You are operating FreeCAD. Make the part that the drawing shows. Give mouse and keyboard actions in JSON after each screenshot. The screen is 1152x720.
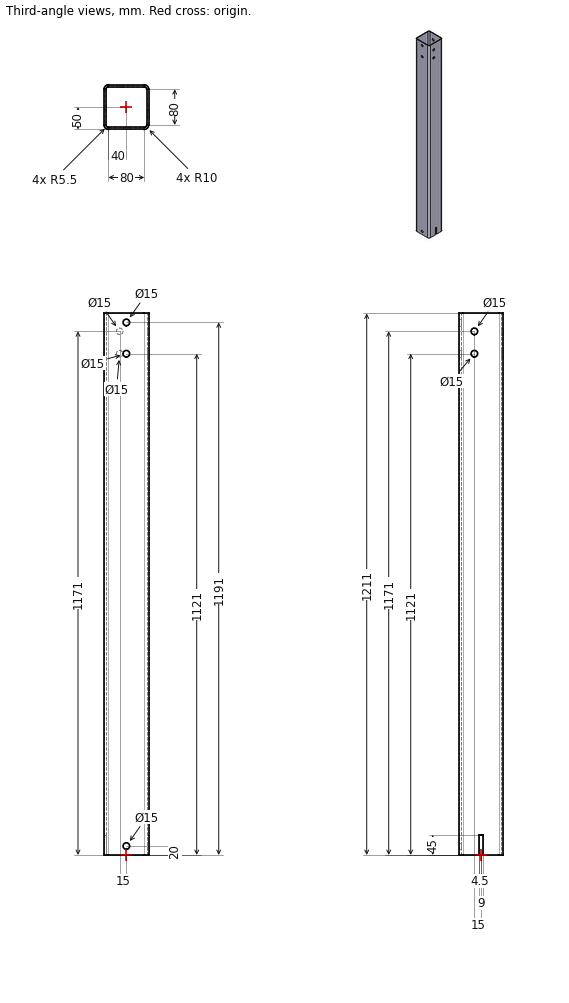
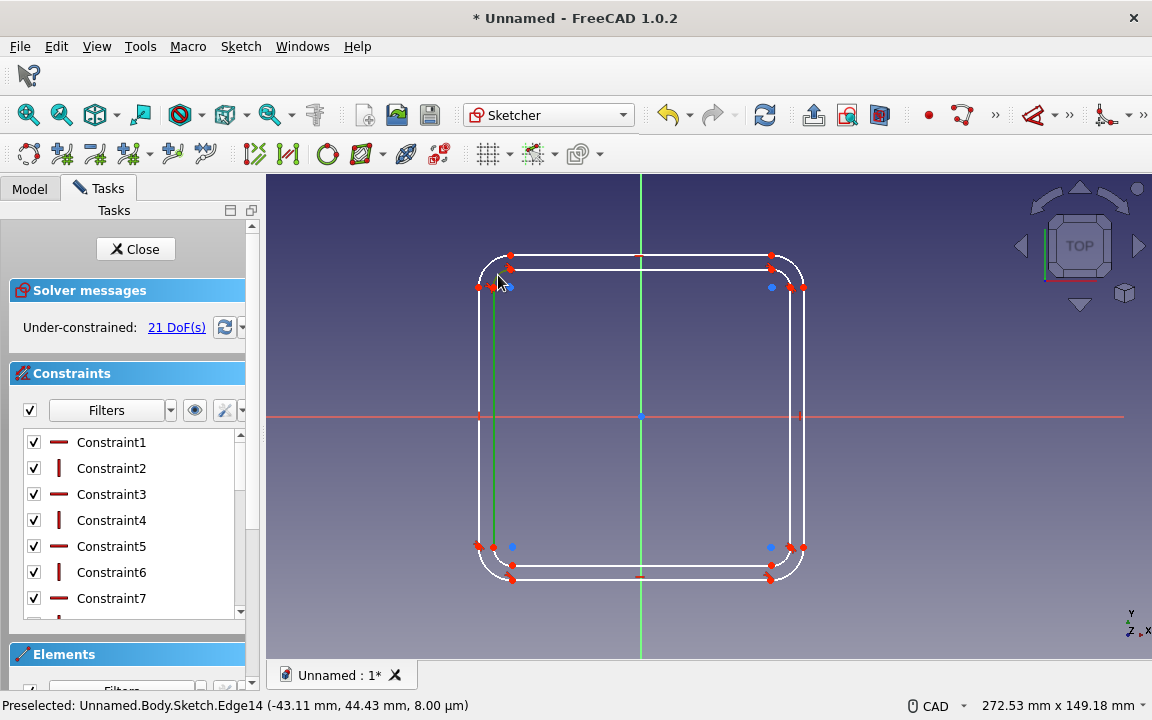
{"action": "key", "text": "t"}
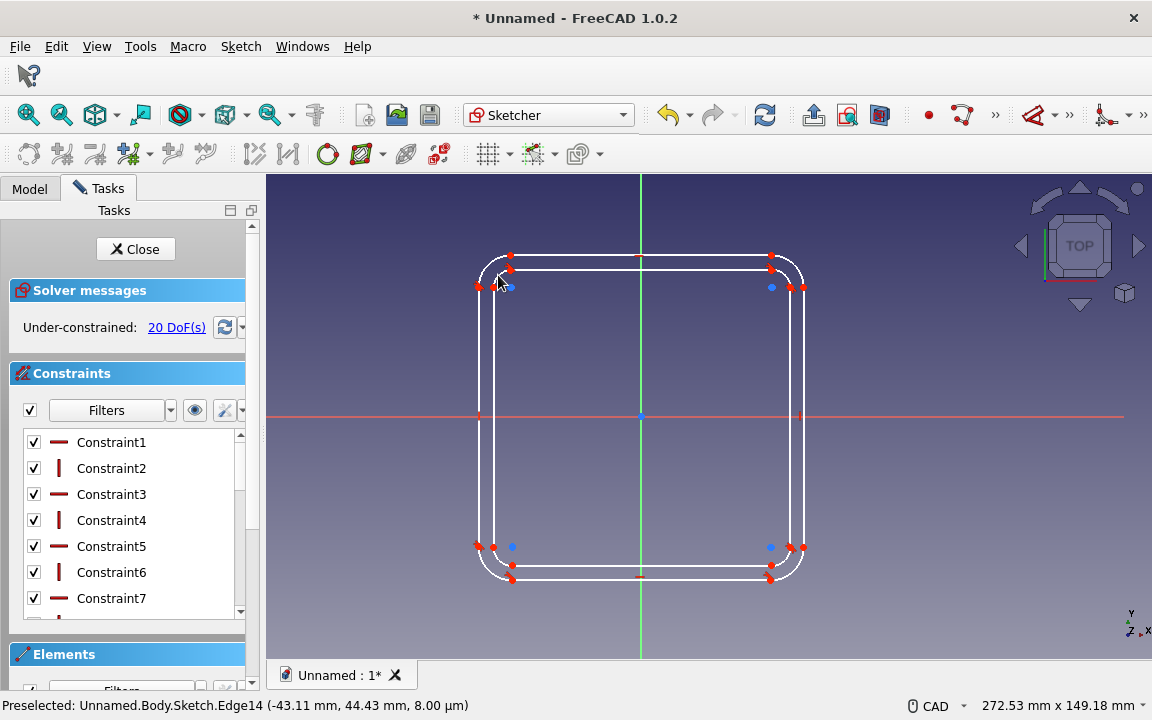
{"action": "left_click", "coordinate": [589, 270]}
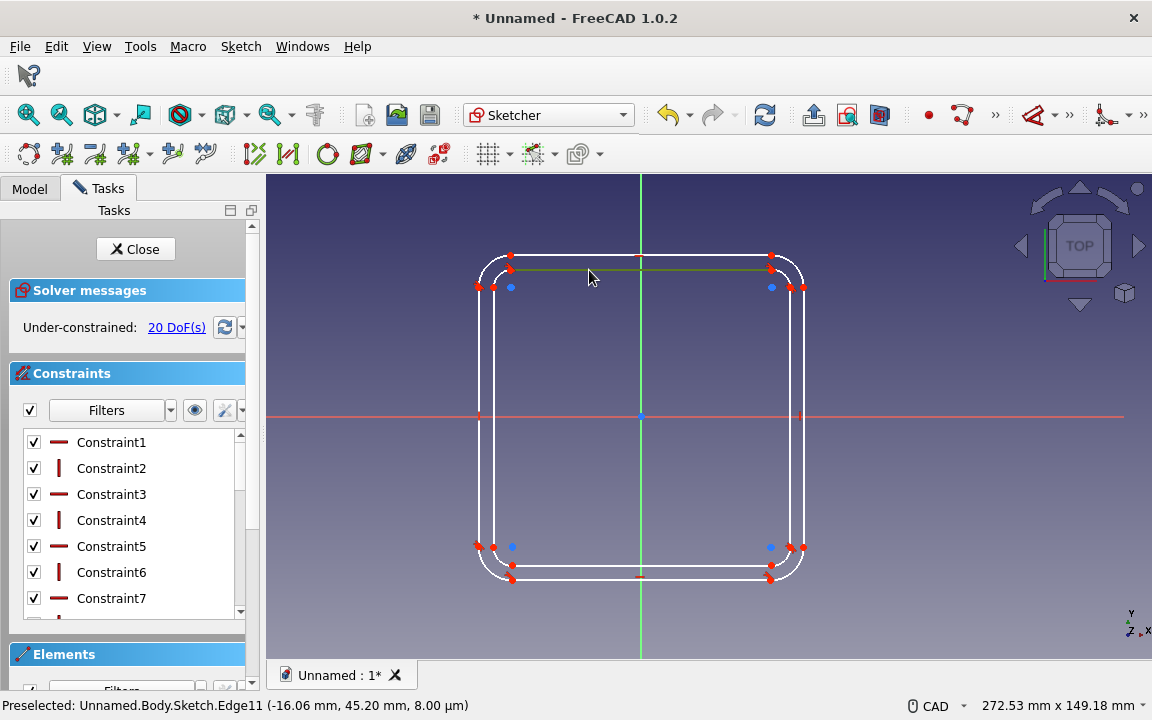
{"action": "left_click", "coordinate": [499, 276]}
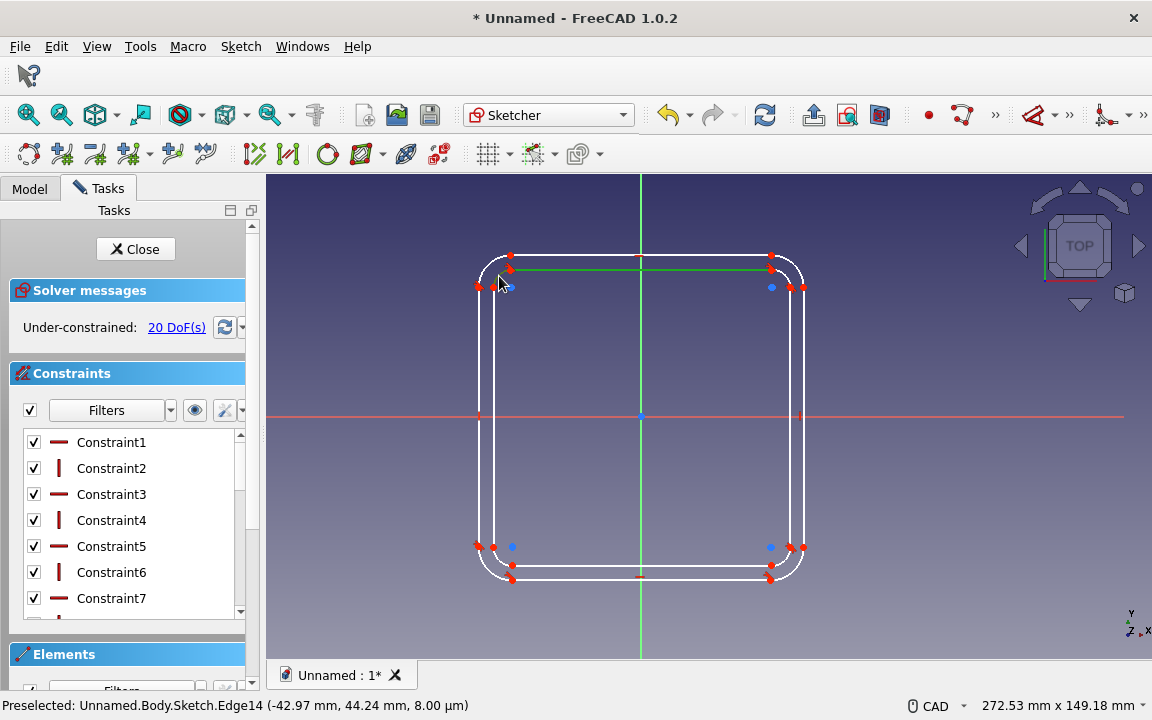
{"action": "key", "text": "t"}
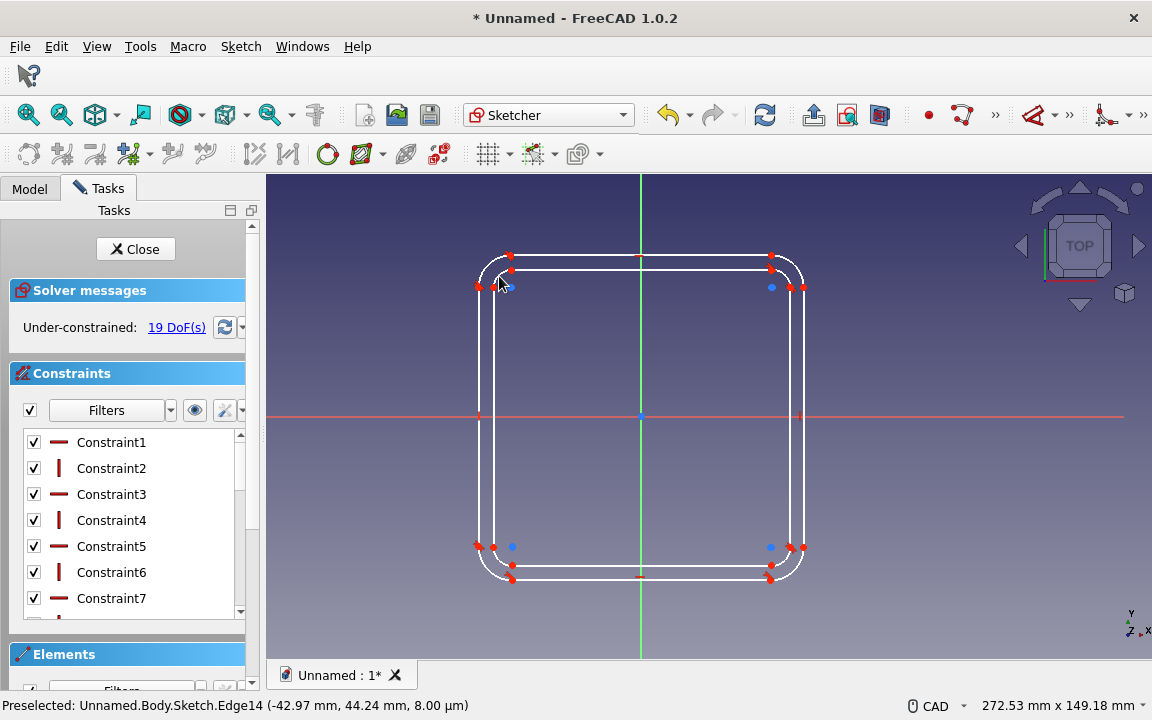
{"action": "left_click", "coordinate": [590, 270]}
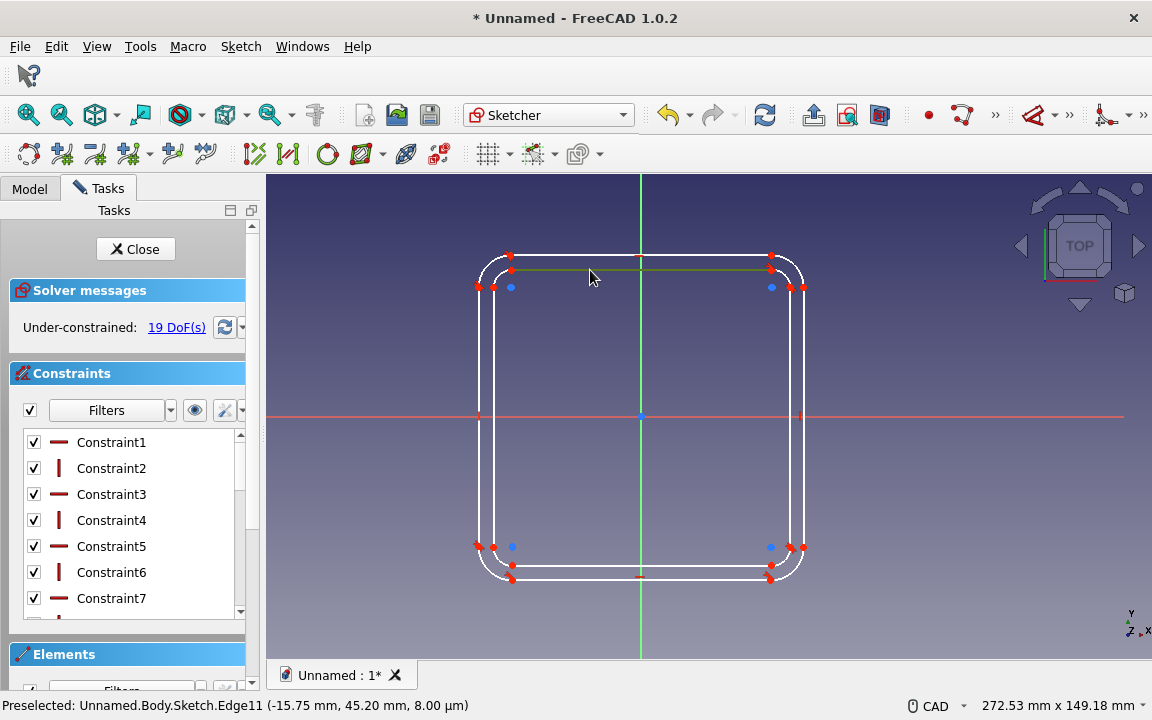
{"action": "left_click", "coordinate": [785, 275]}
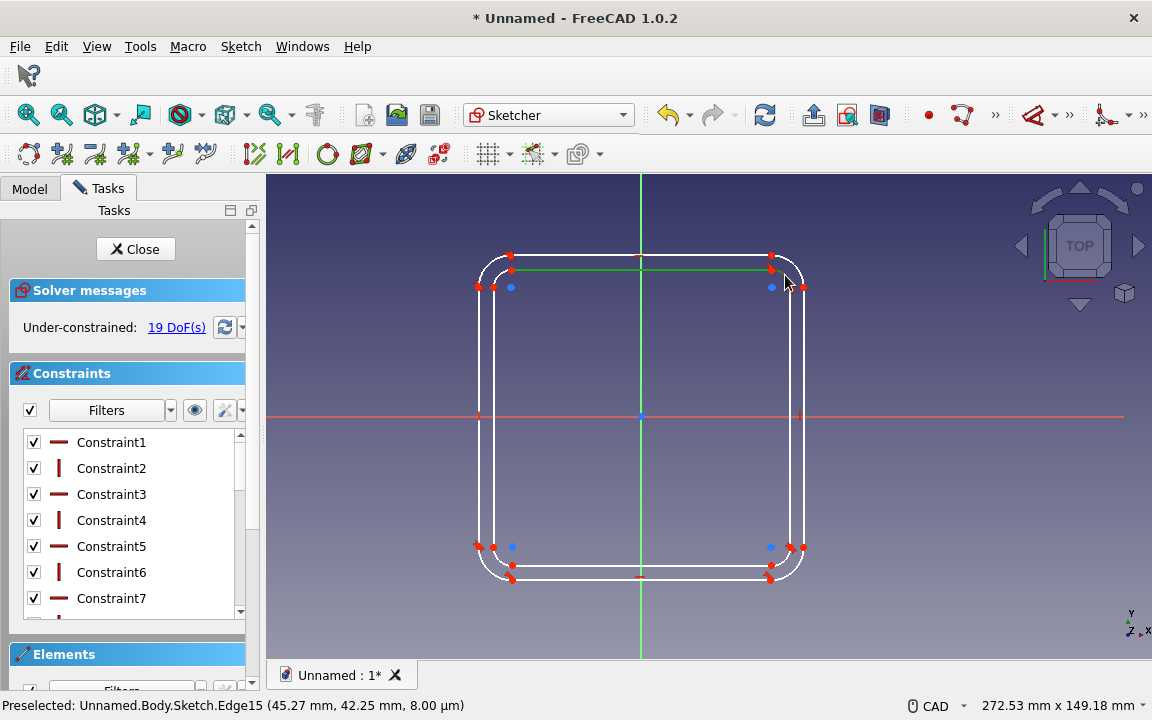
{"action": "key", "text": "t"}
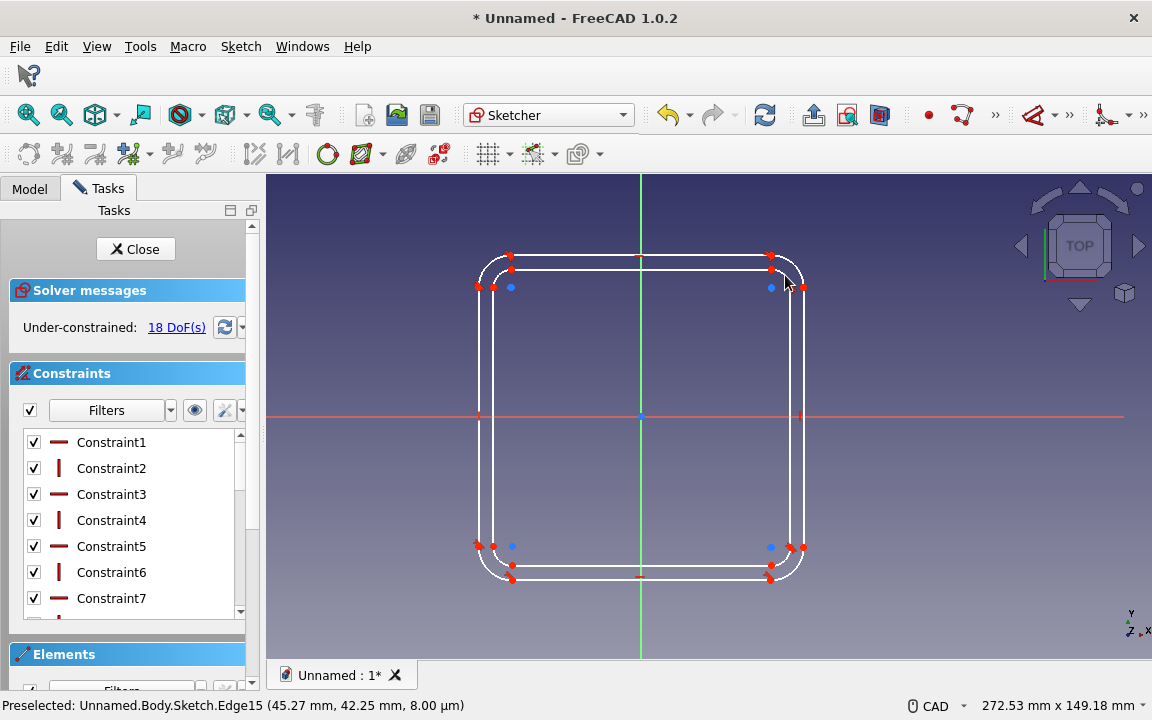
{"action": "left_click", "coordinate": [790, 366]}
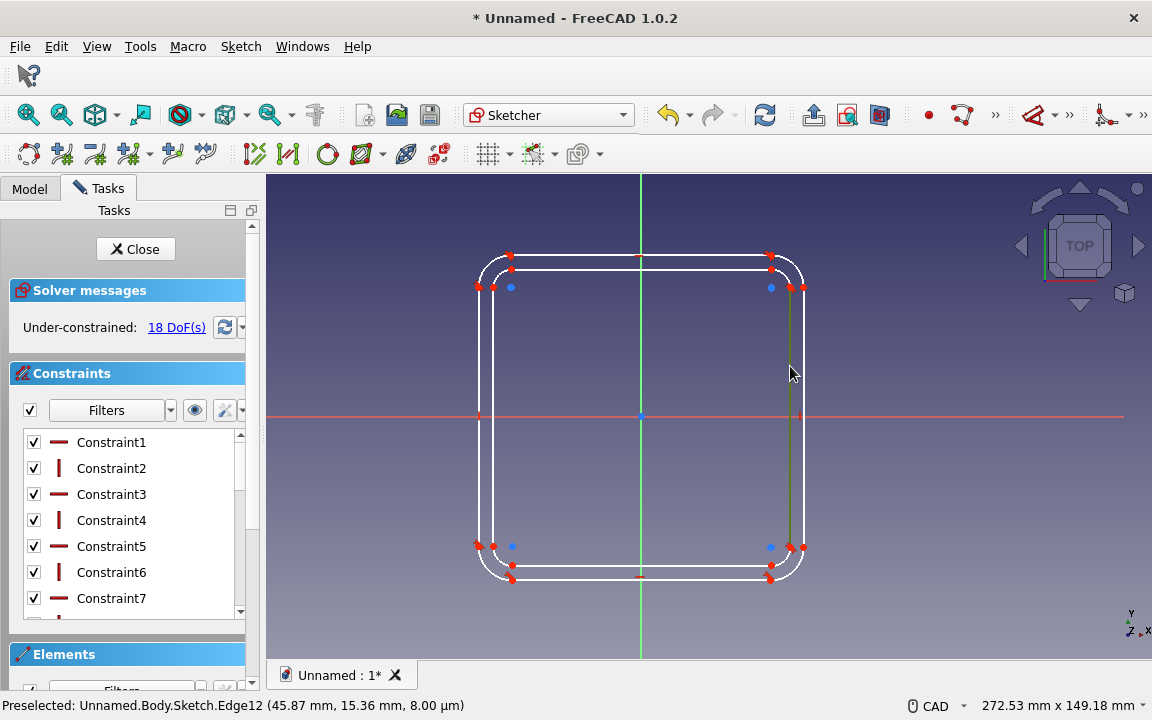
{"action": "left_click", "coordinate": [785, 275]}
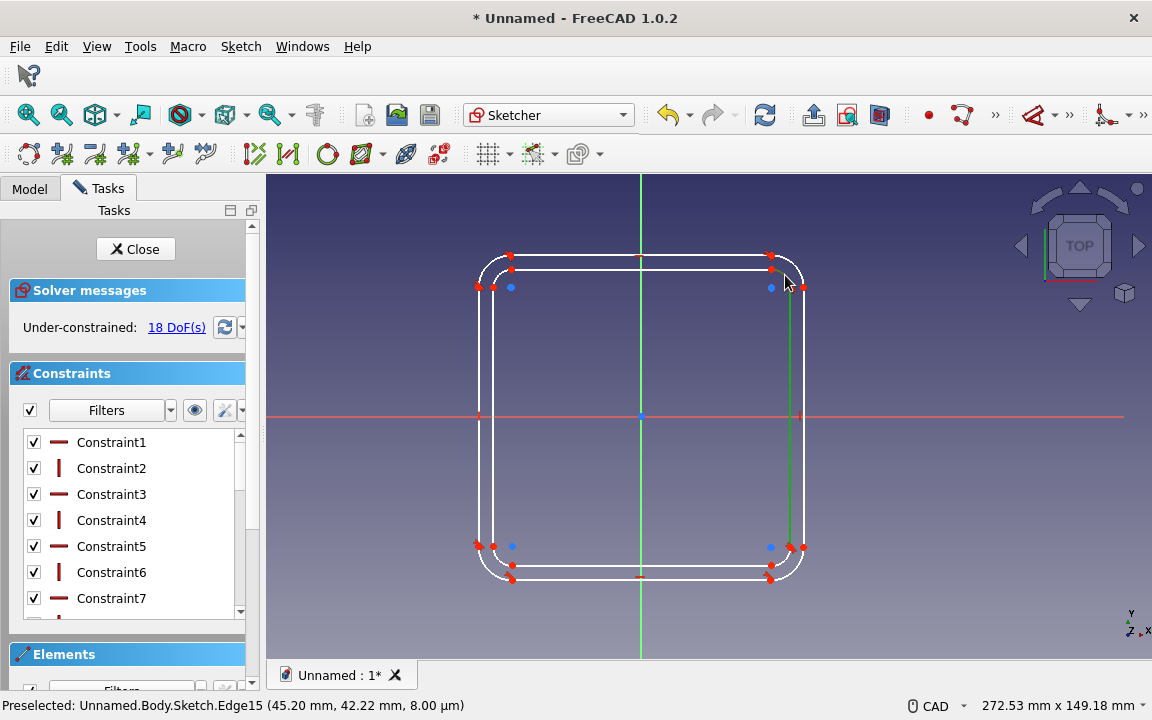
{"action": "key", "text": "t"}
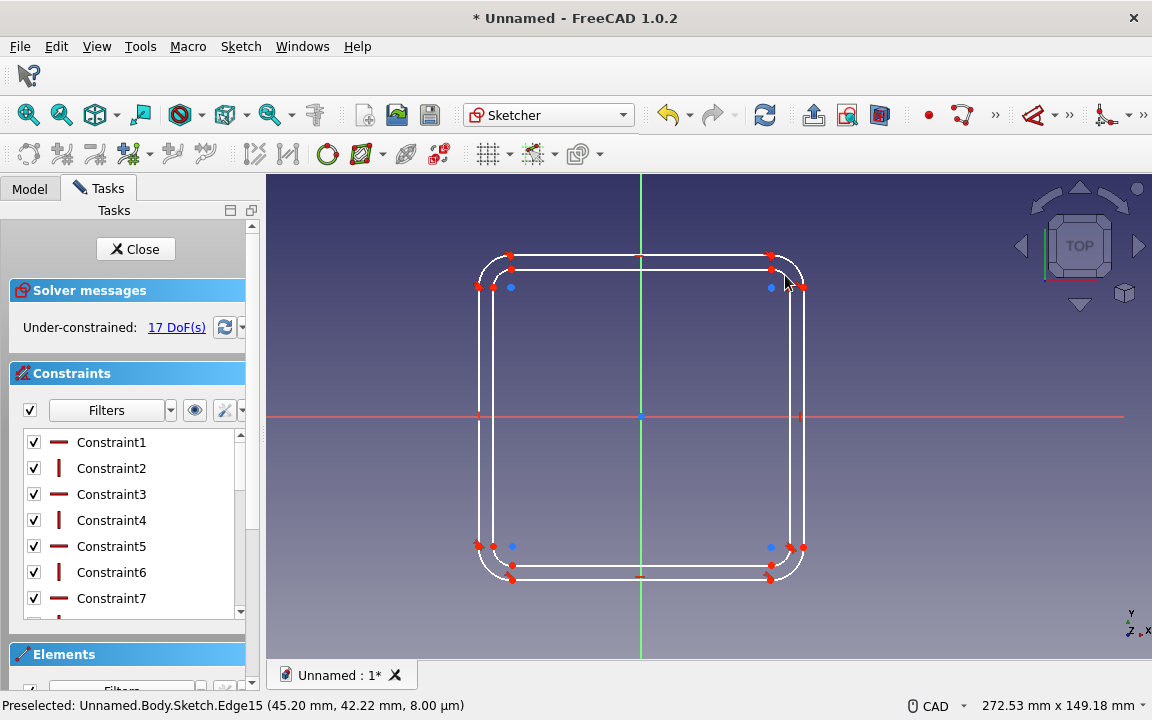
{"action": "left_click", "coordinate": [790, 366]}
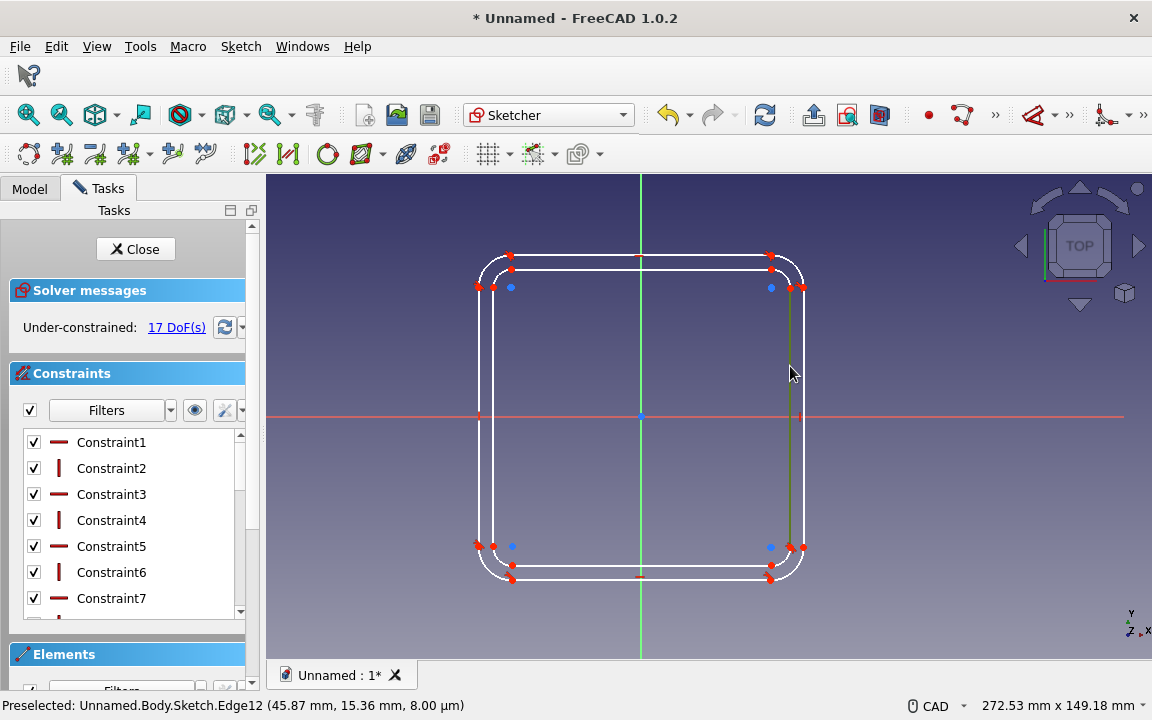
{"action": "left_click", "coordinate": [785, 561]}